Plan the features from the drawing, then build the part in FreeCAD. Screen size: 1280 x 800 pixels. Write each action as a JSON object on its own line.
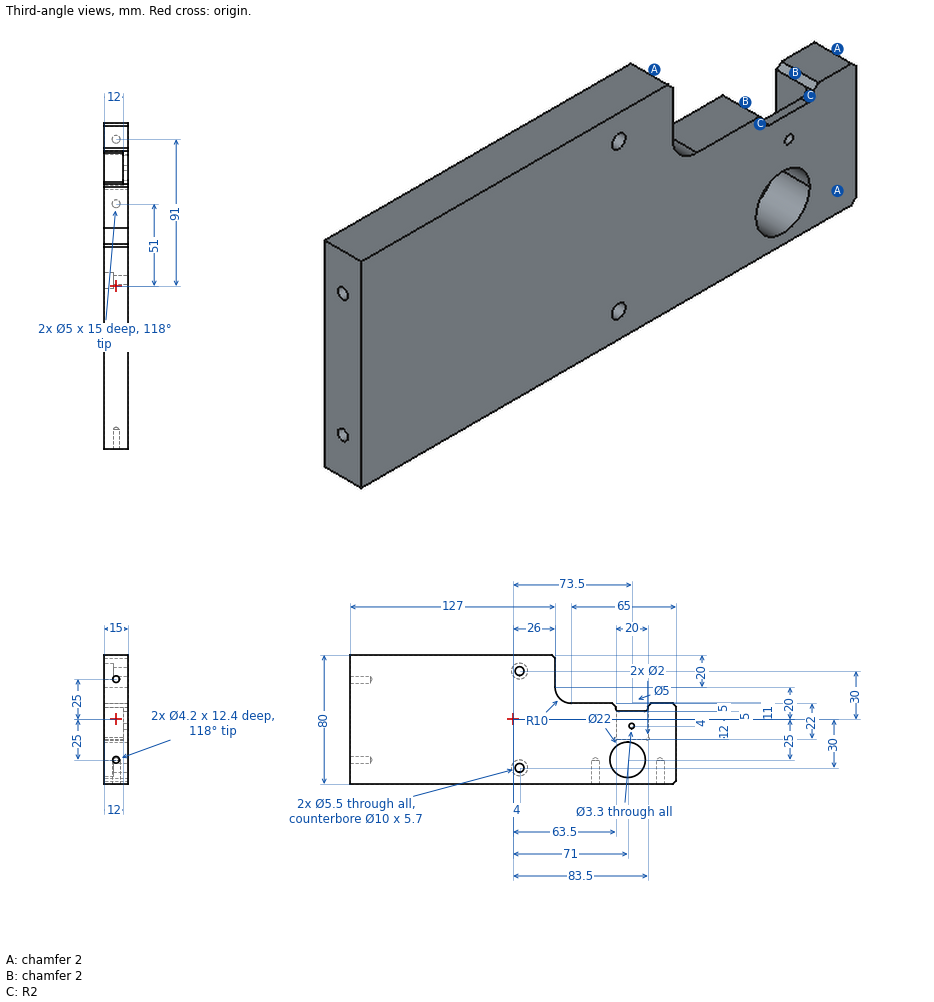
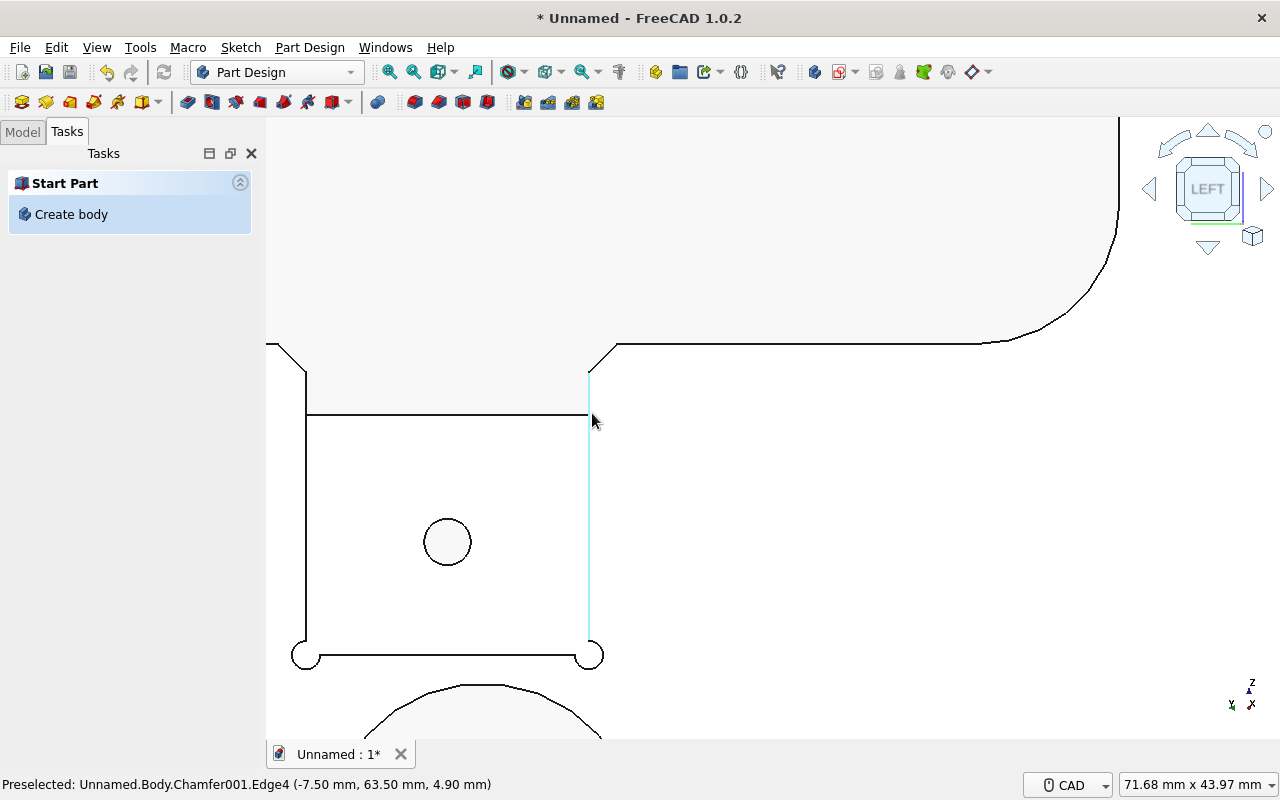
{"action": "left_click", "coordinate": [390, 72]}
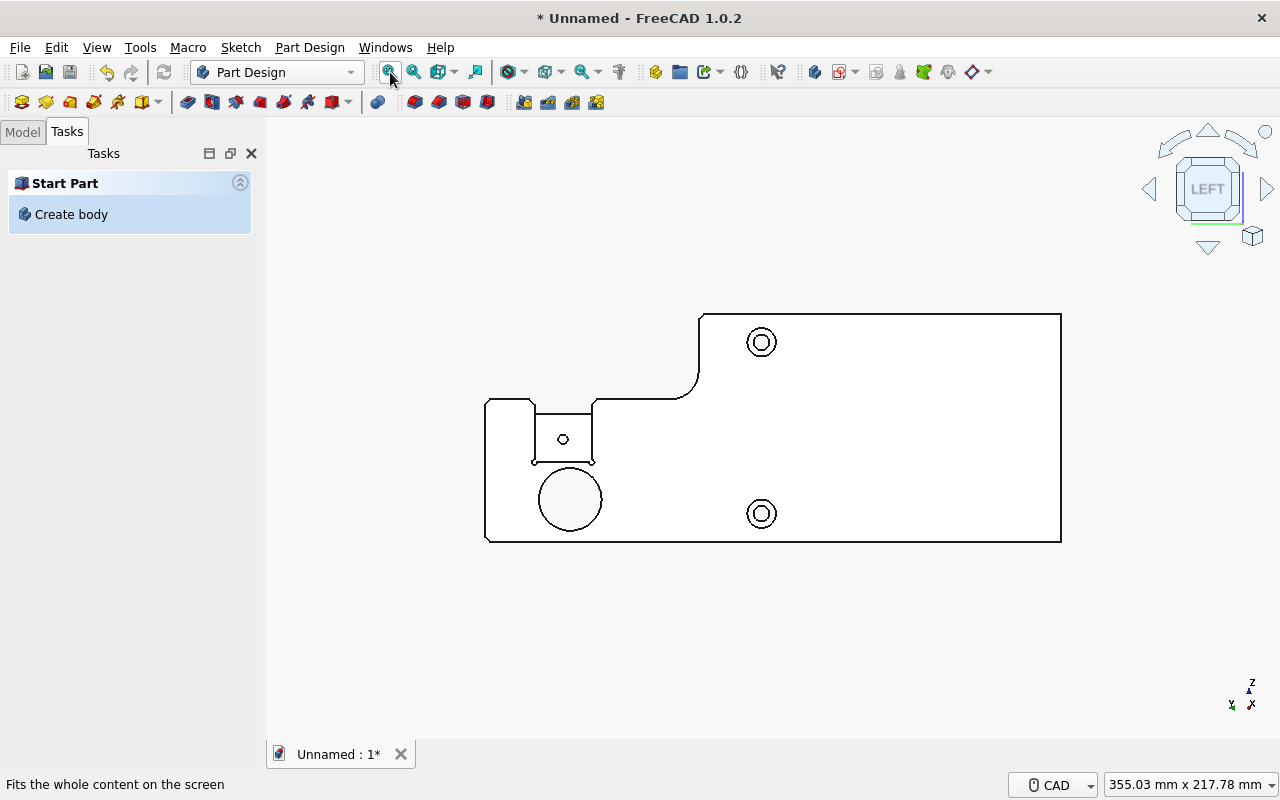
{"action": "key", "text": "v 3"}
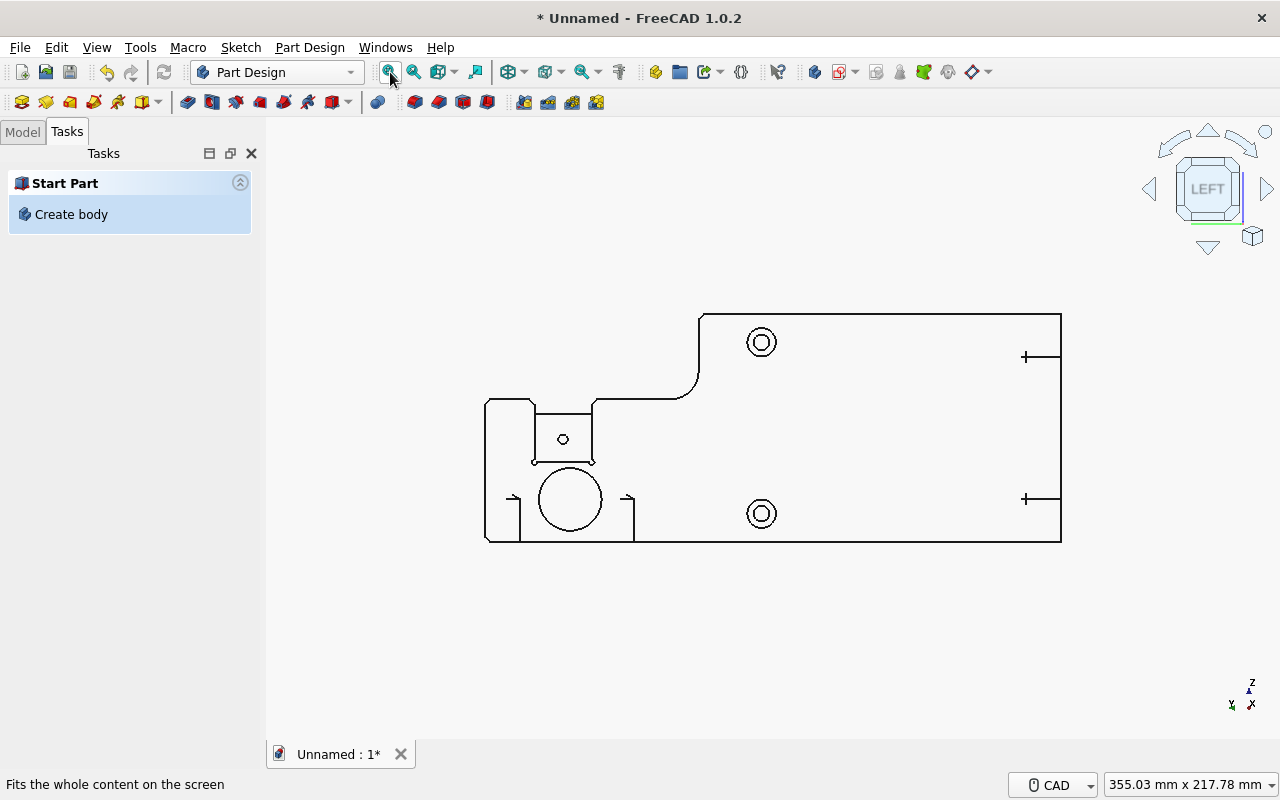
{"action": "key", "text": "0"}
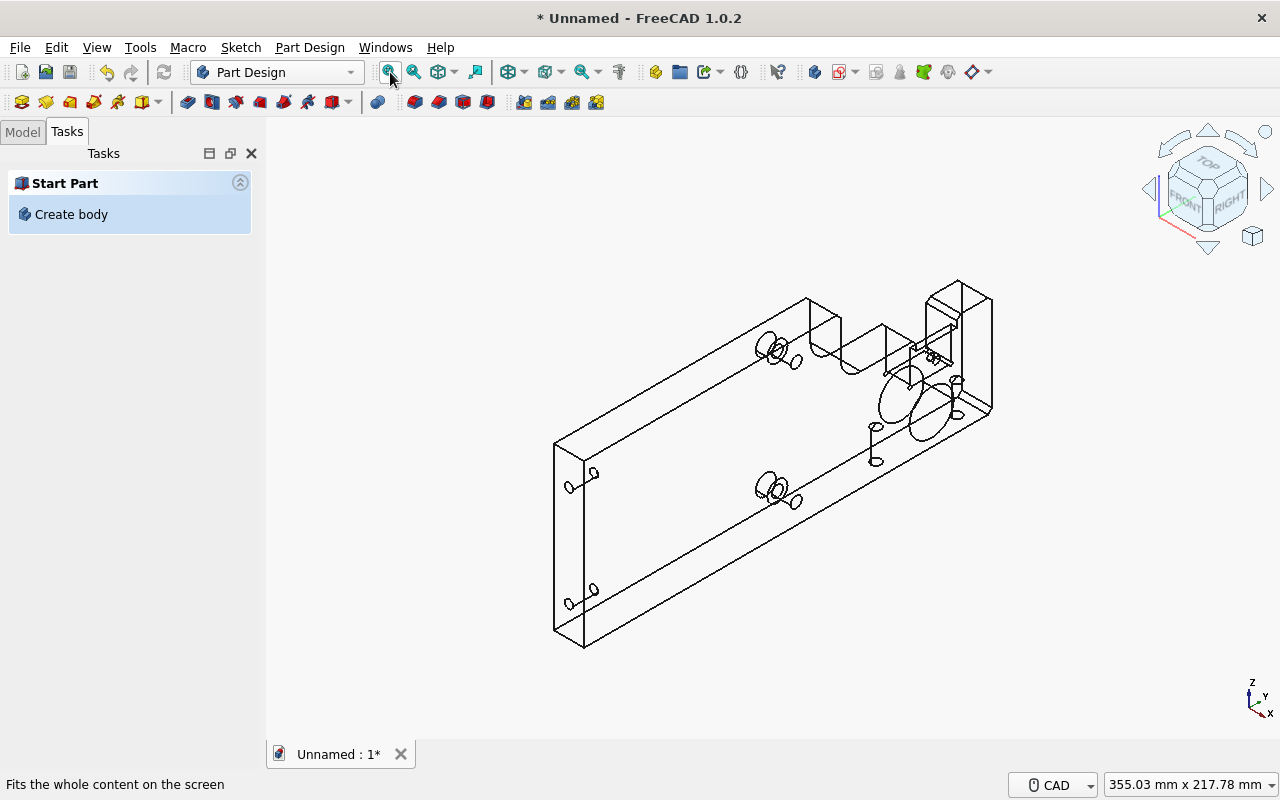
{"action": "scroll", "coordinate": [913, 348], "scroll_direction": "up", "scroll_amount": 8}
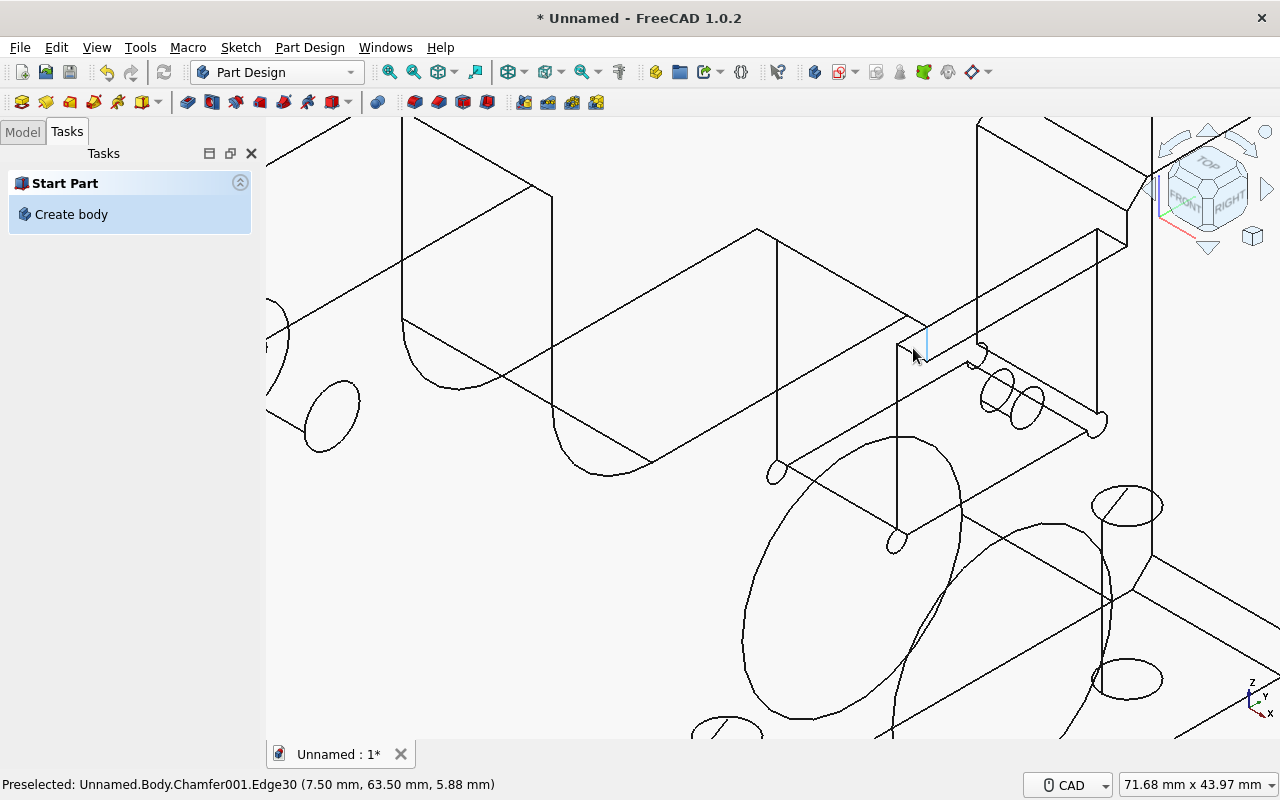
{"action": "left_click", "coordinate": [912, 352]}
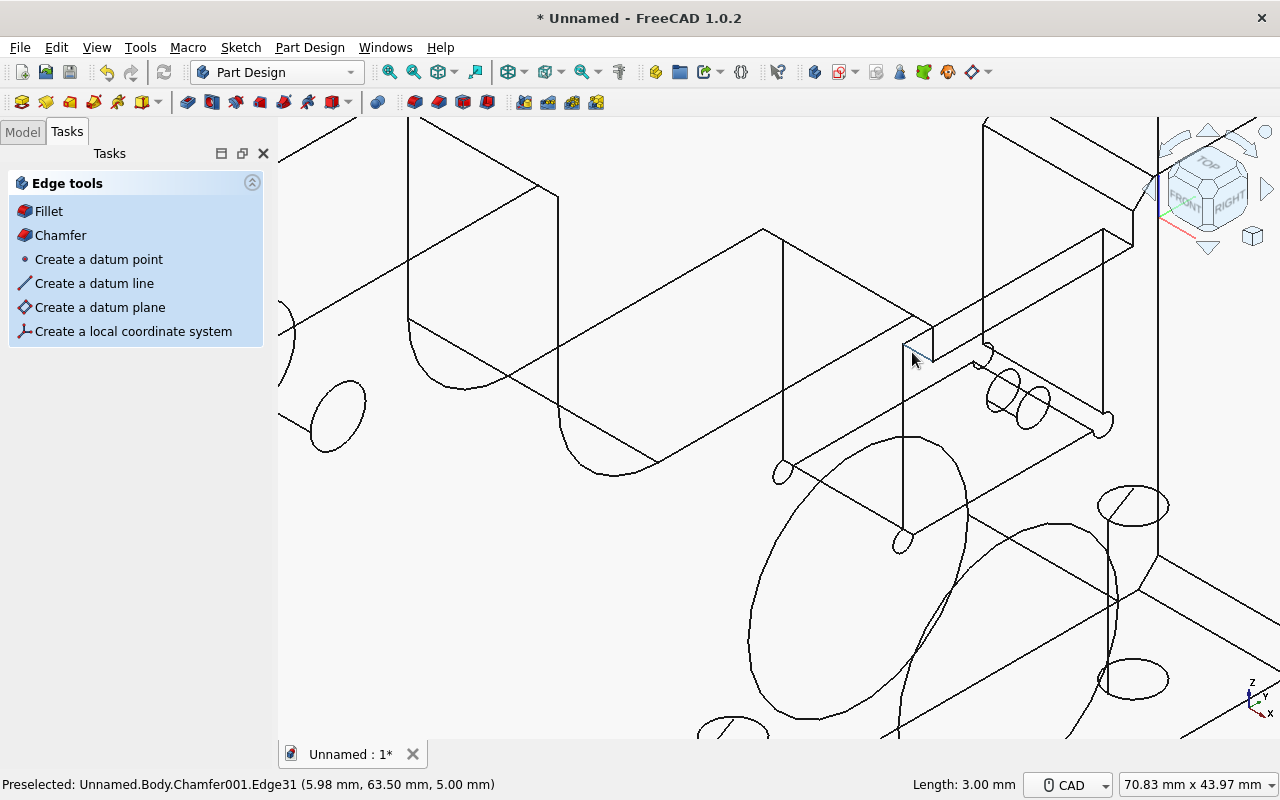
{"action": "left_click", "coordinate": [1115, 235], "text": "ctrl"}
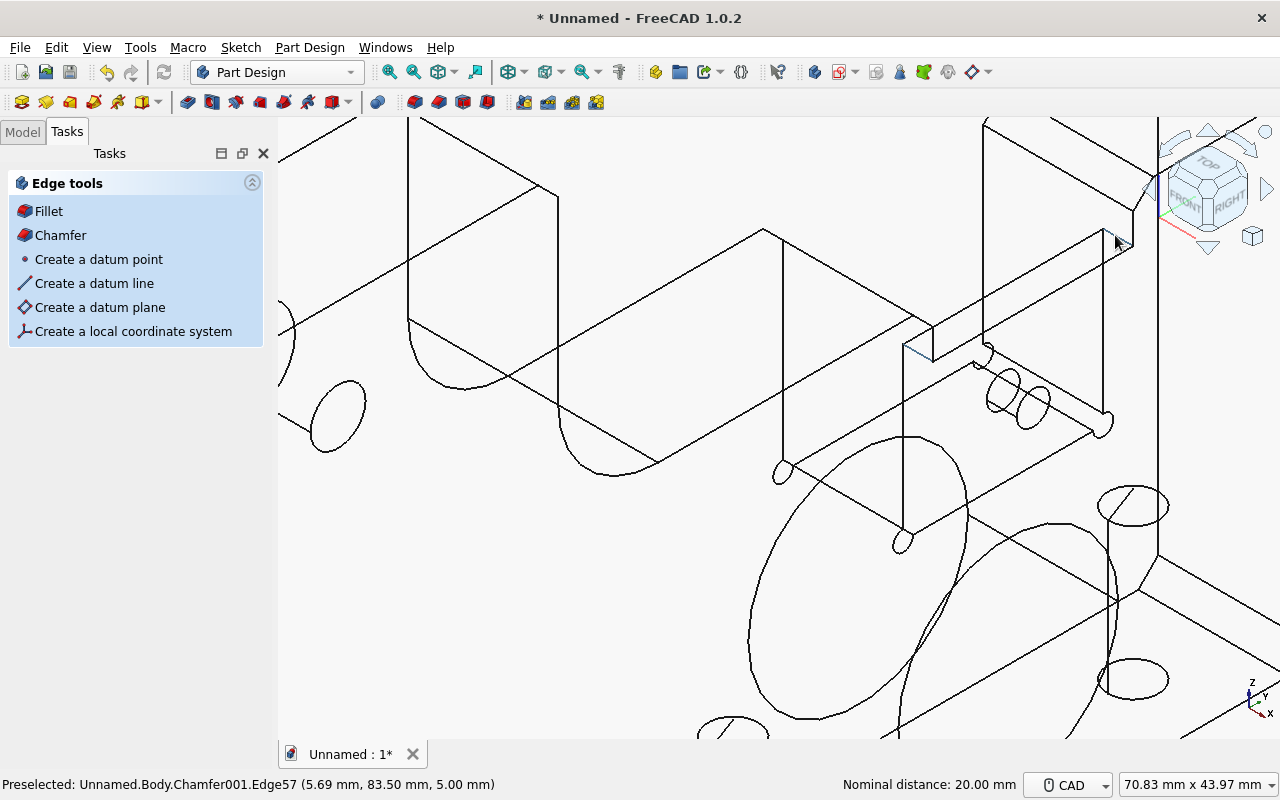
{"action": "key", "text": "v 1"}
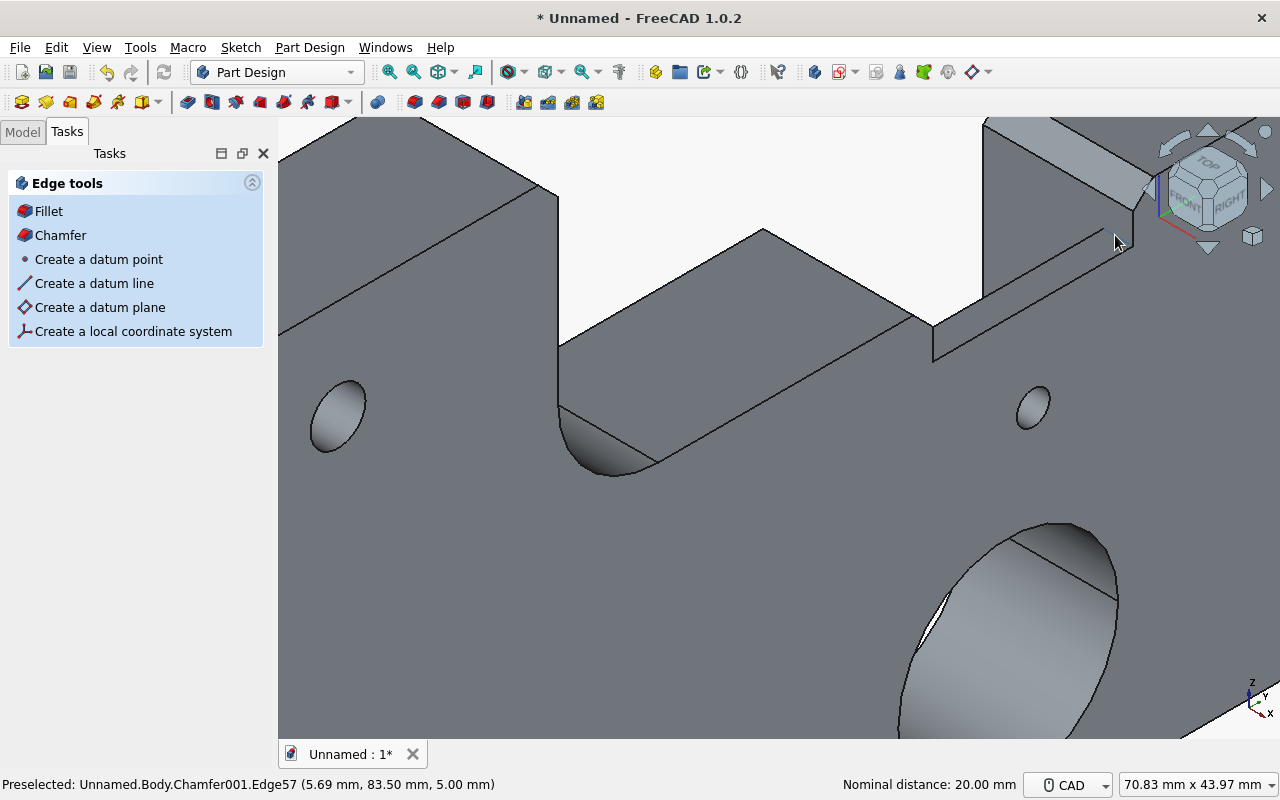
{"action": "left_click", "coordinate": [416, 102]}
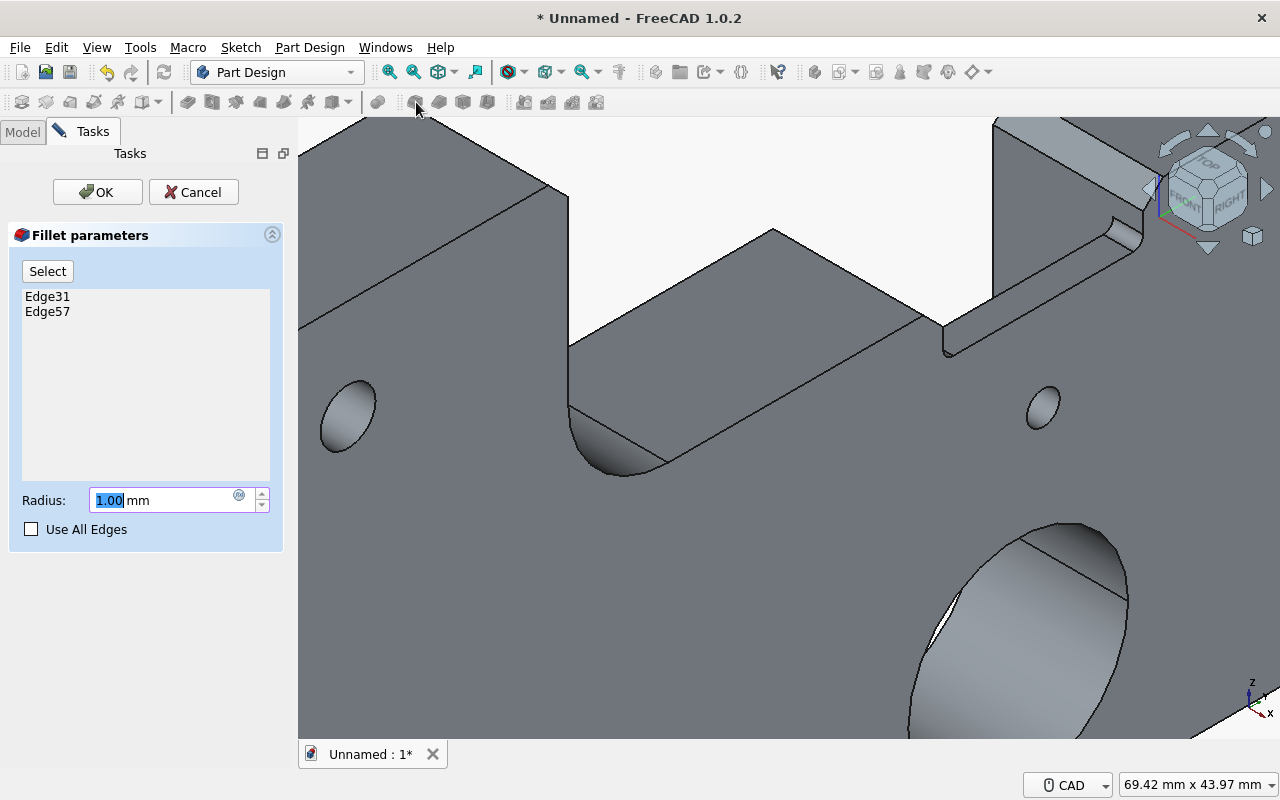
{"action": "type", "text": "2"}
{"action": "key", "text": "Tab"}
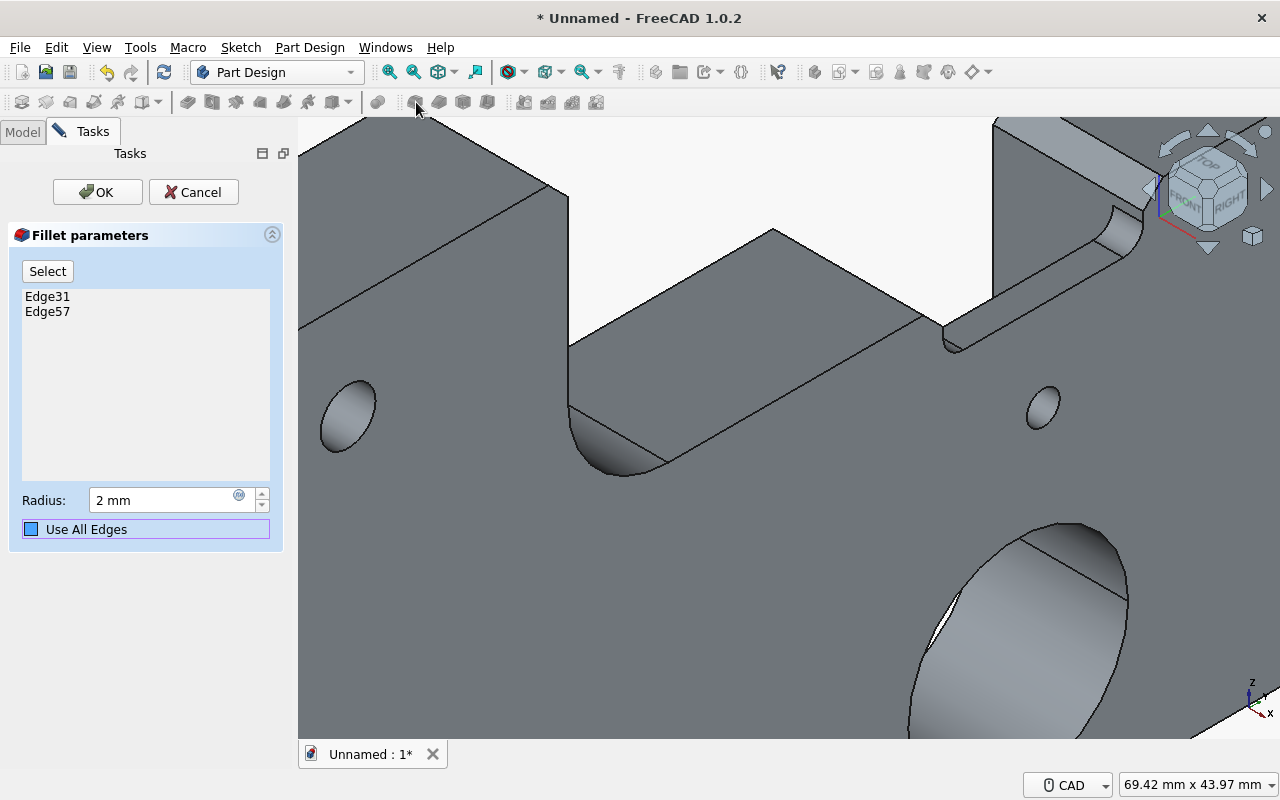
{"action": "left_click", "coordinate": [98, 192]}